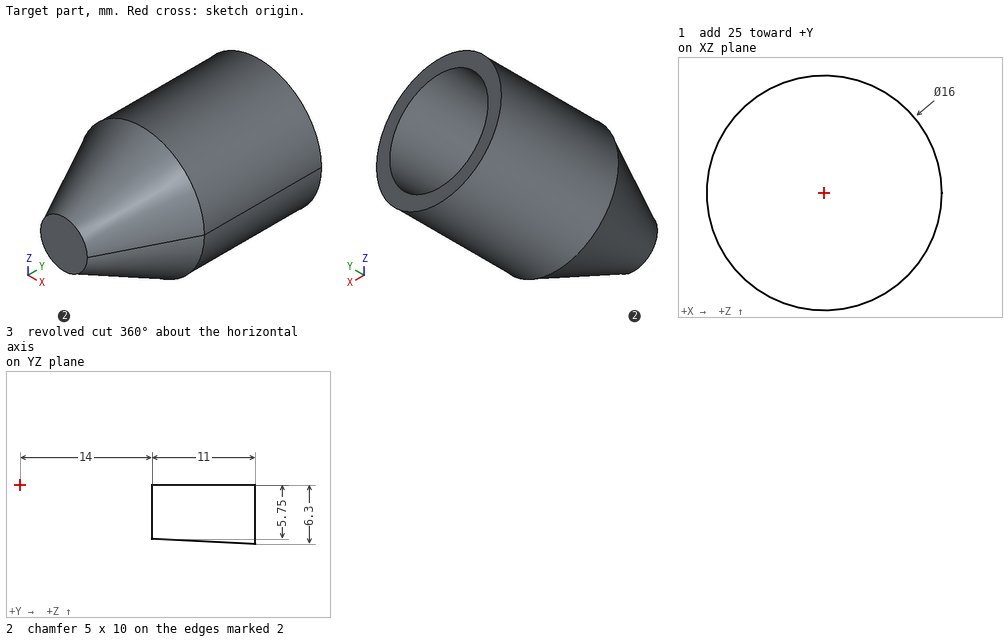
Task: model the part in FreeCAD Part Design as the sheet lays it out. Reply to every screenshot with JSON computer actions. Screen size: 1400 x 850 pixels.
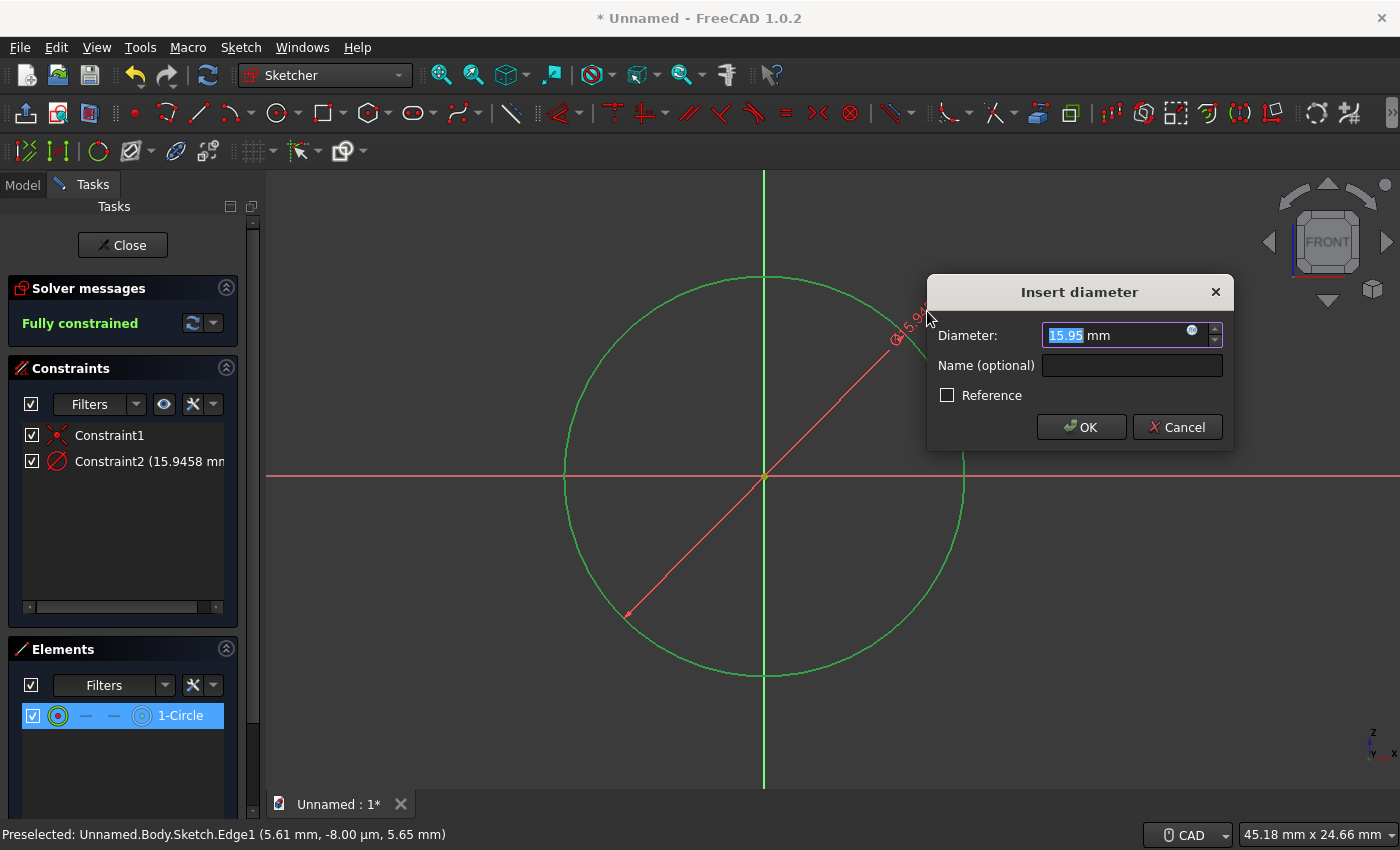
{"action": "type", "text": "16"}
{"action": "key", "text": "Return"}
{"action": "key", "text": "Escape"}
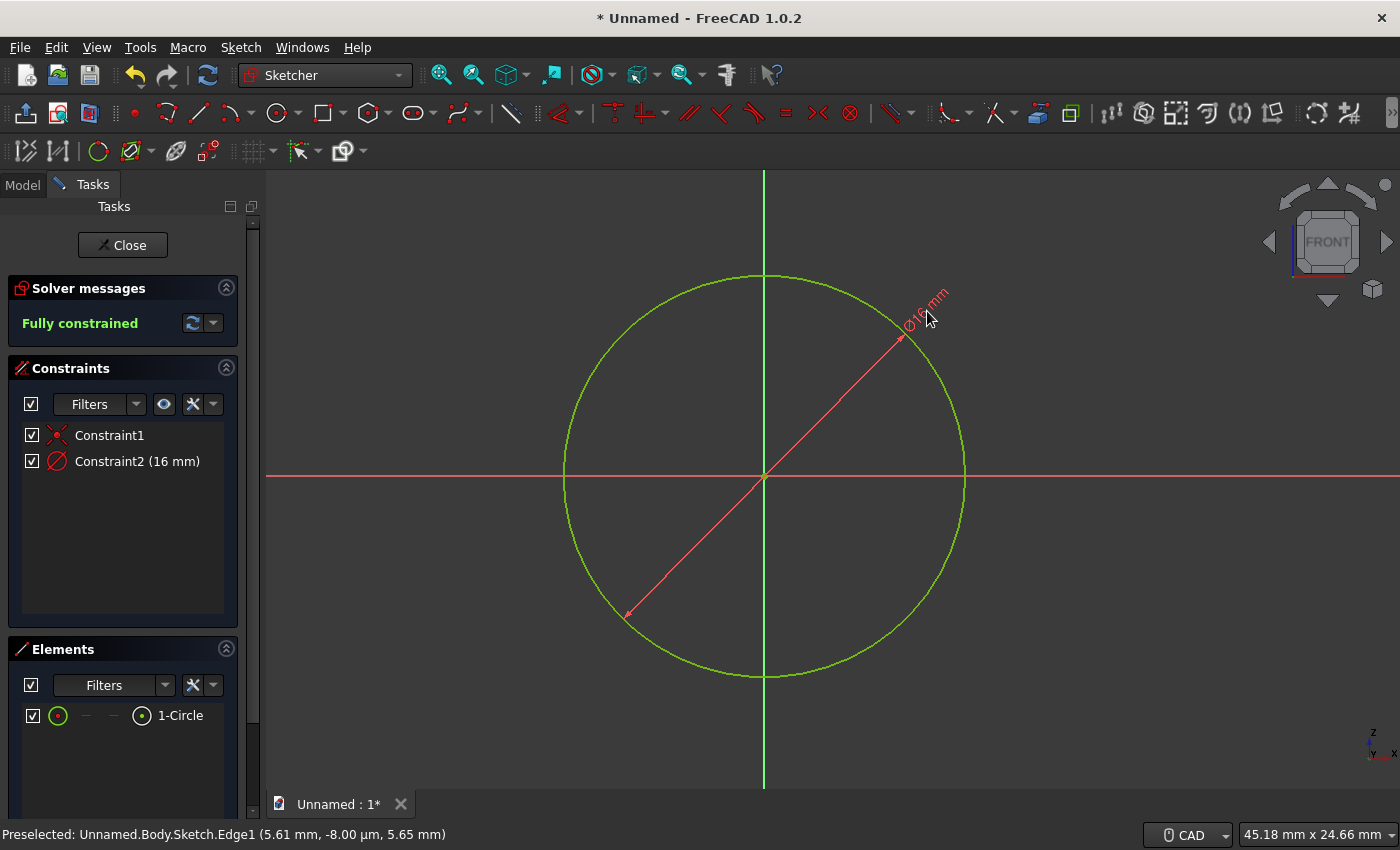
{"action": "left_click", "coordinate": [123, 245]}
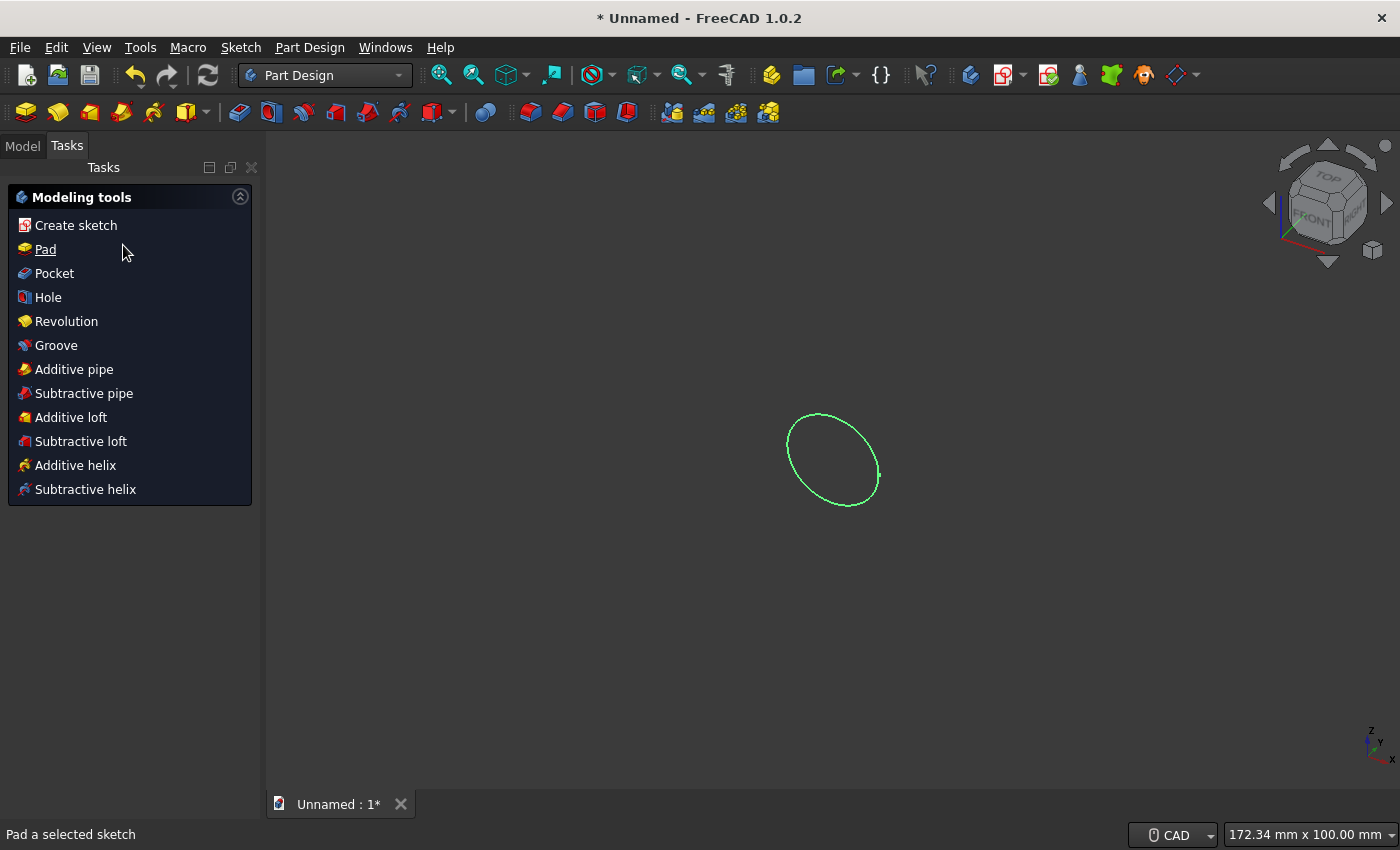
{"action": "left_click", "coordinate": [26, 112]}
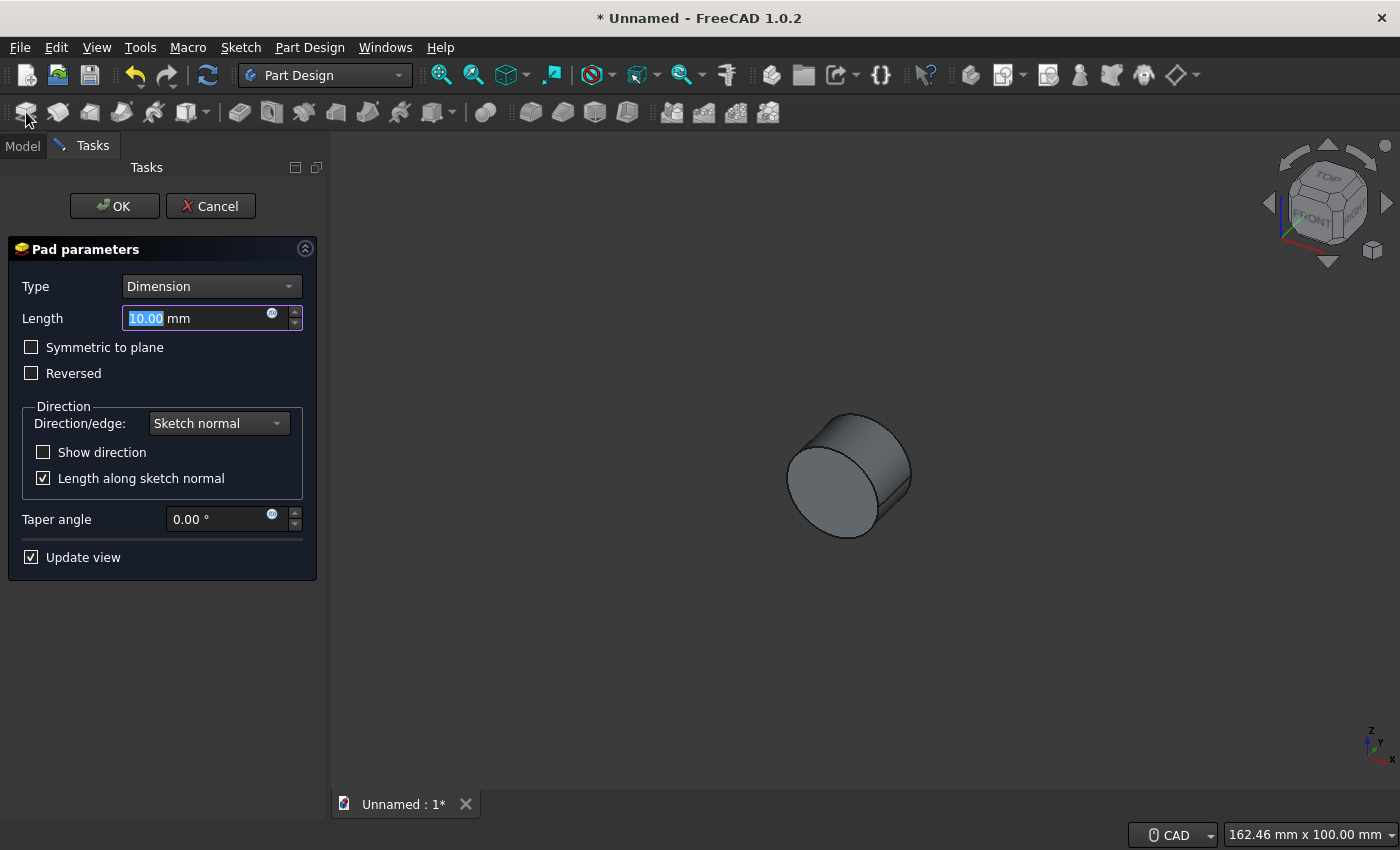
{"action": "type", "text": "25"}
{"action": "key", "text": "Tab"}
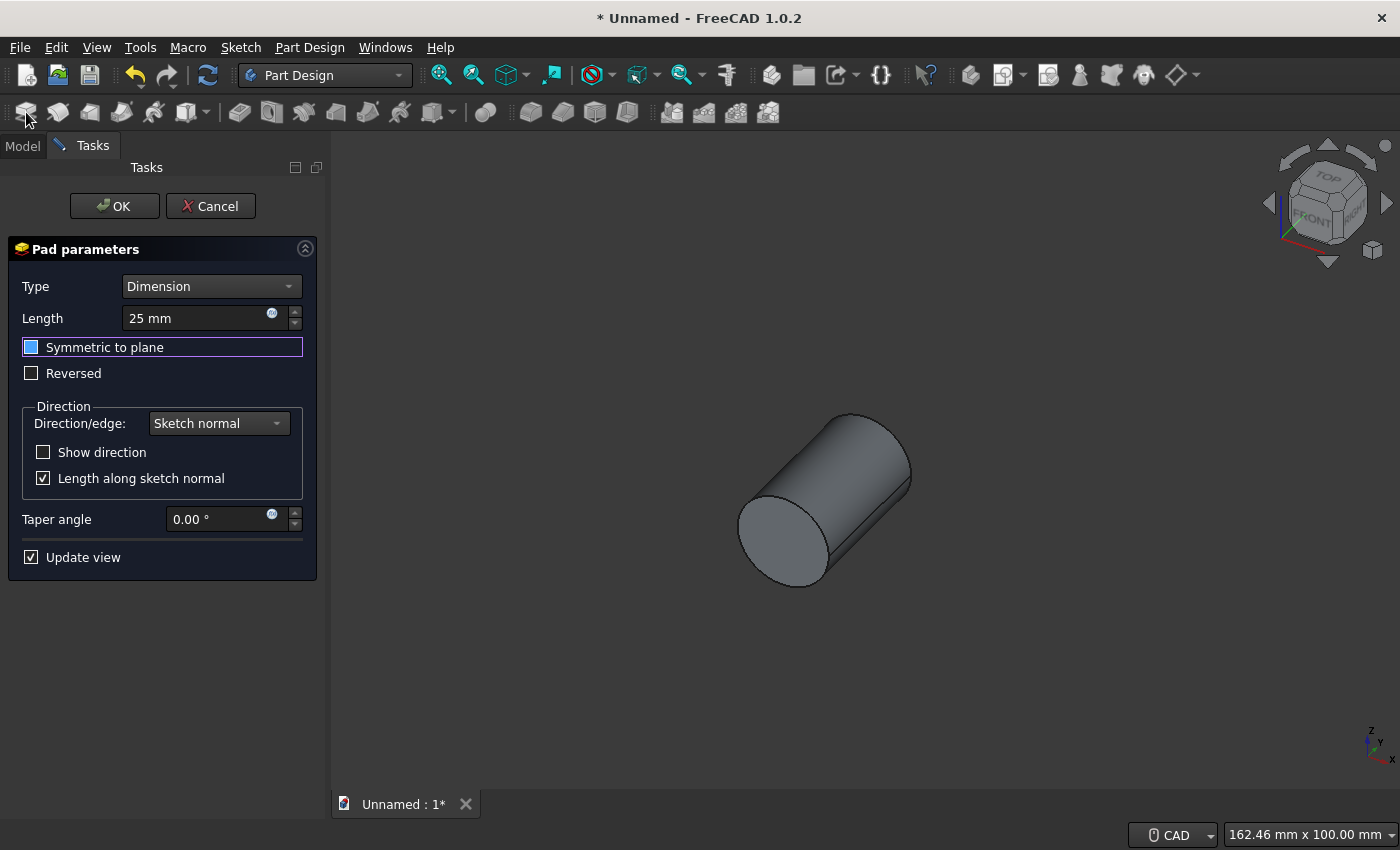
{"action": "left_click", "coordinate": [30, 373]}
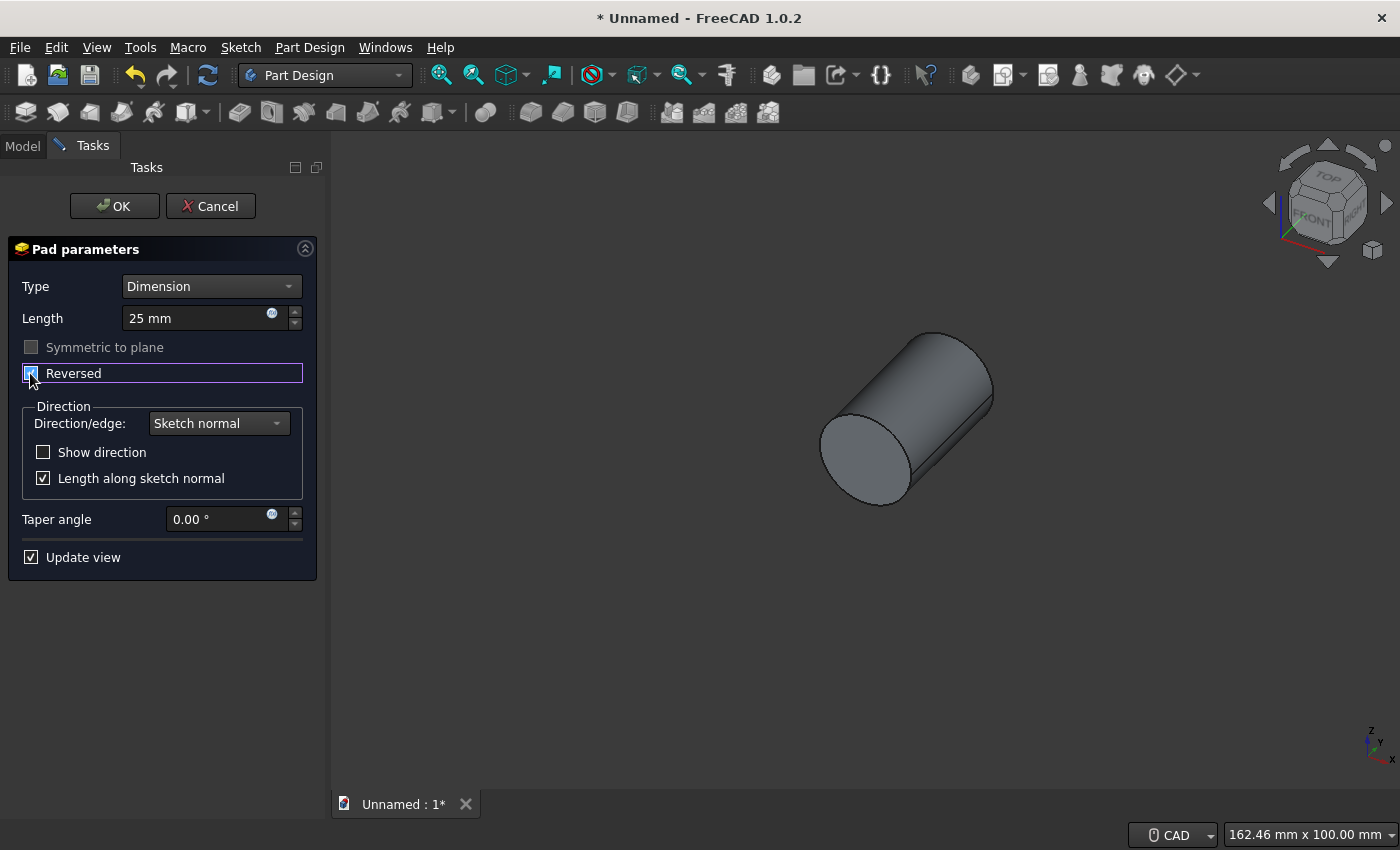
{"action": "left_click", "coordinate": [115, 206]}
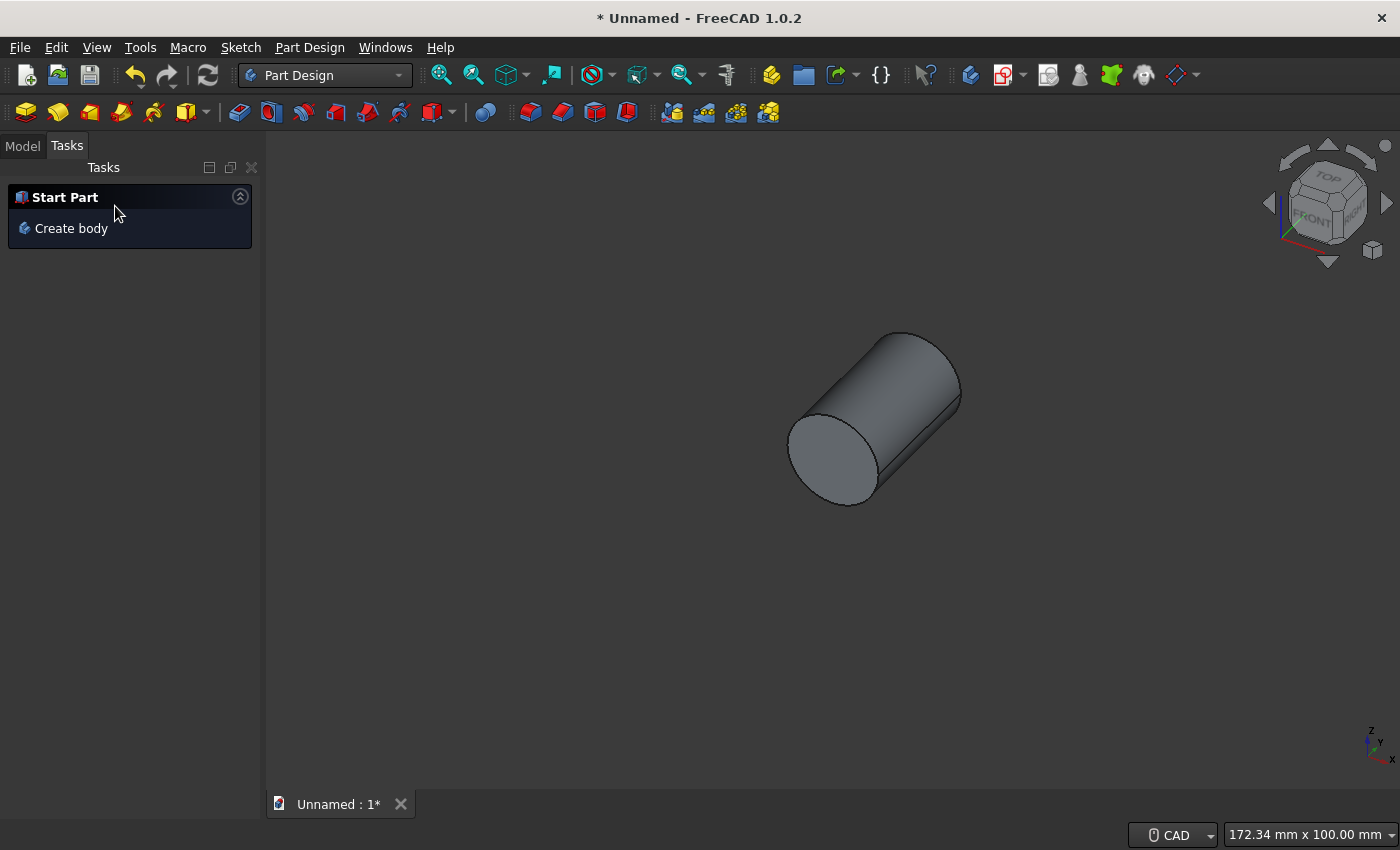
{"action": "left_click", "coordinate": [442, 76]}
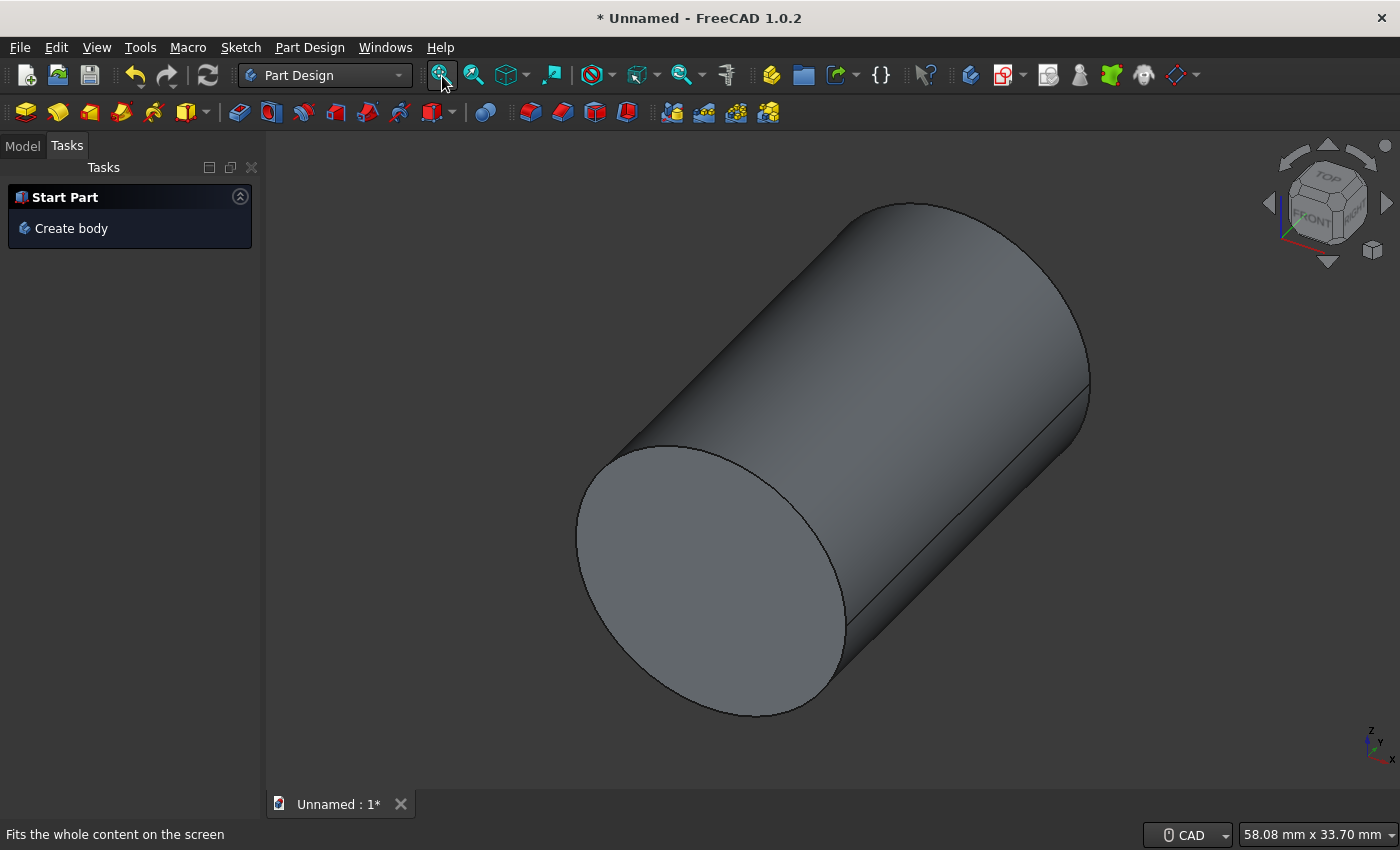
{"action": "left_click", "coordinate": [669, 445]}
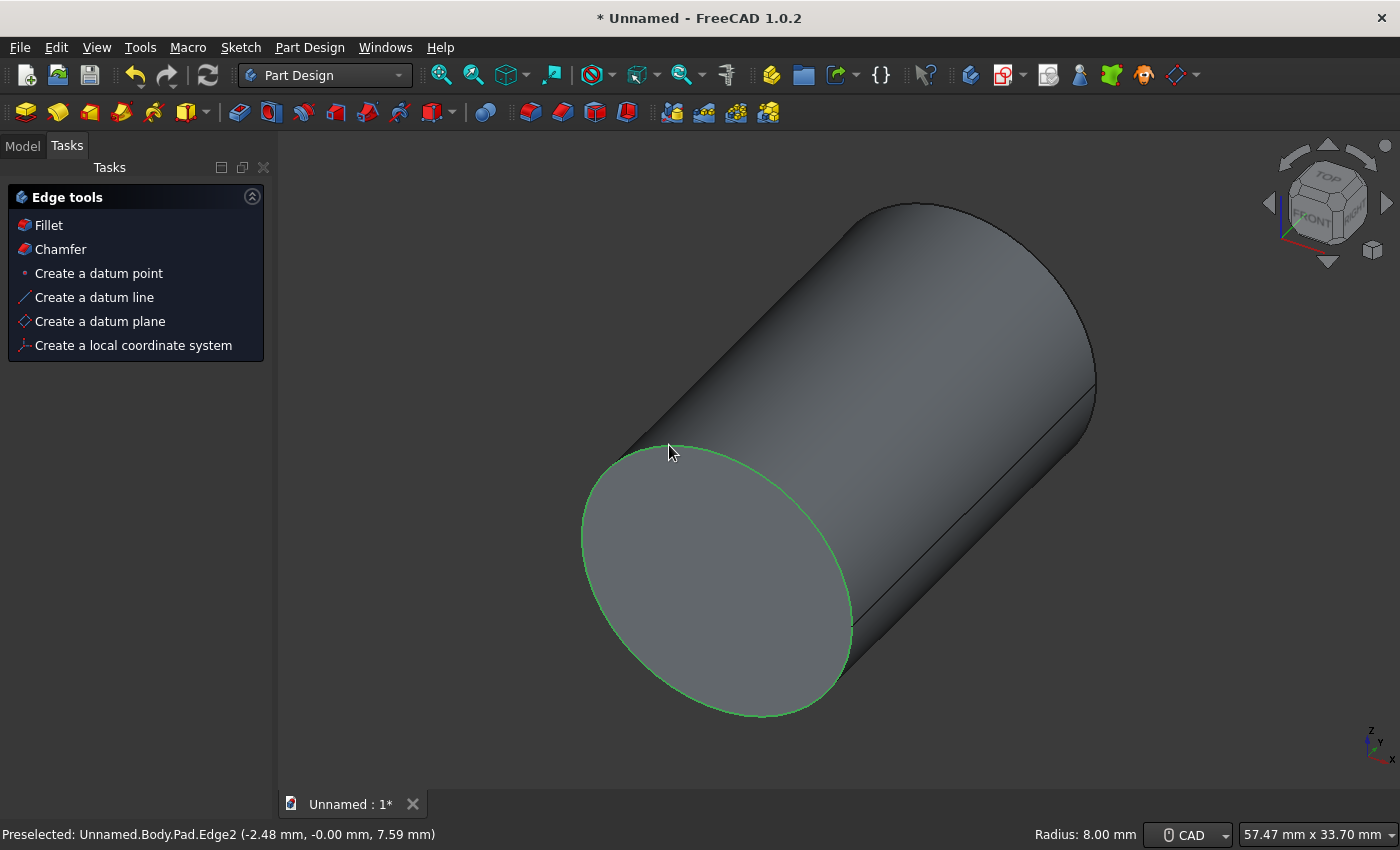
{"action": "left_click", "coordinate": [564, 112]}